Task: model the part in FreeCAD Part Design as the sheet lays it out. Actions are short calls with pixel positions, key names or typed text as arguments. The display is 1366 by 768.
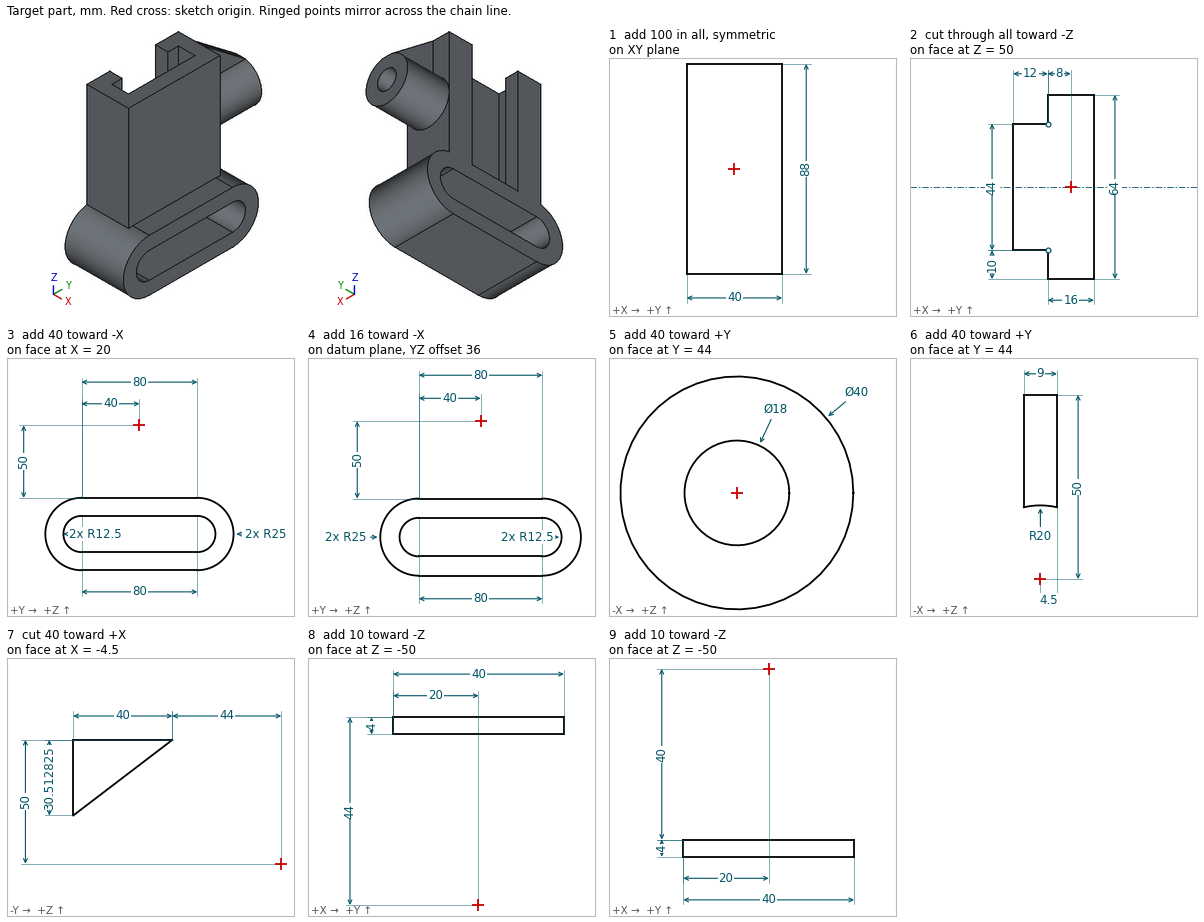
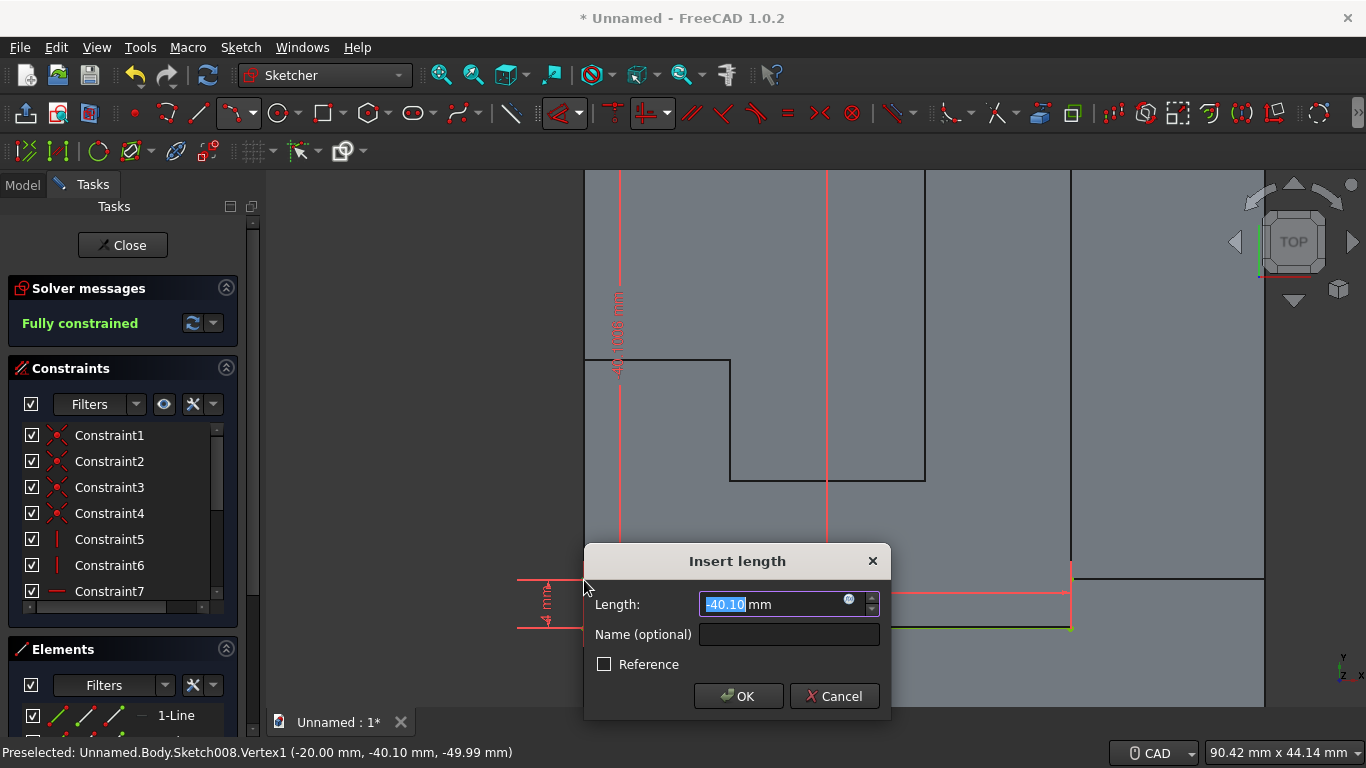
text(-40)
key(Return)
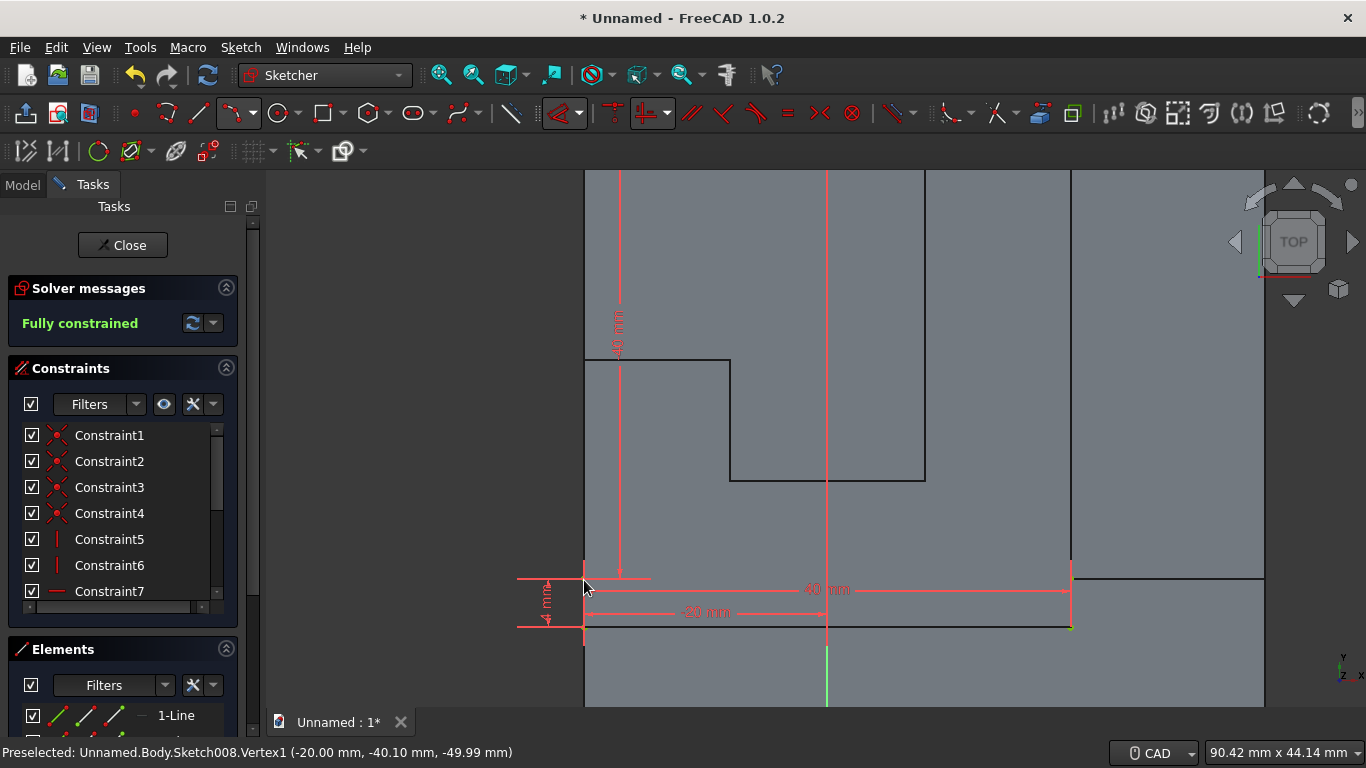
click(123, 245)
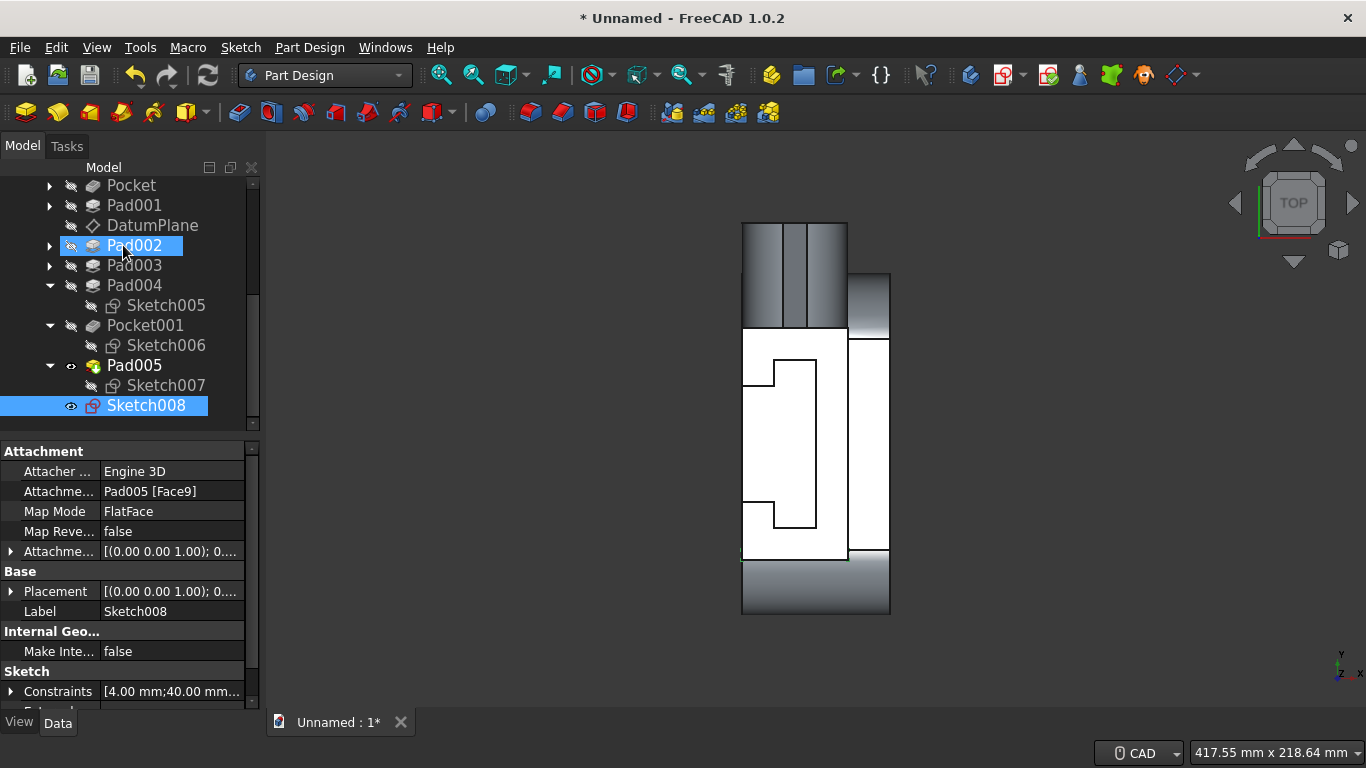
click(26, 112)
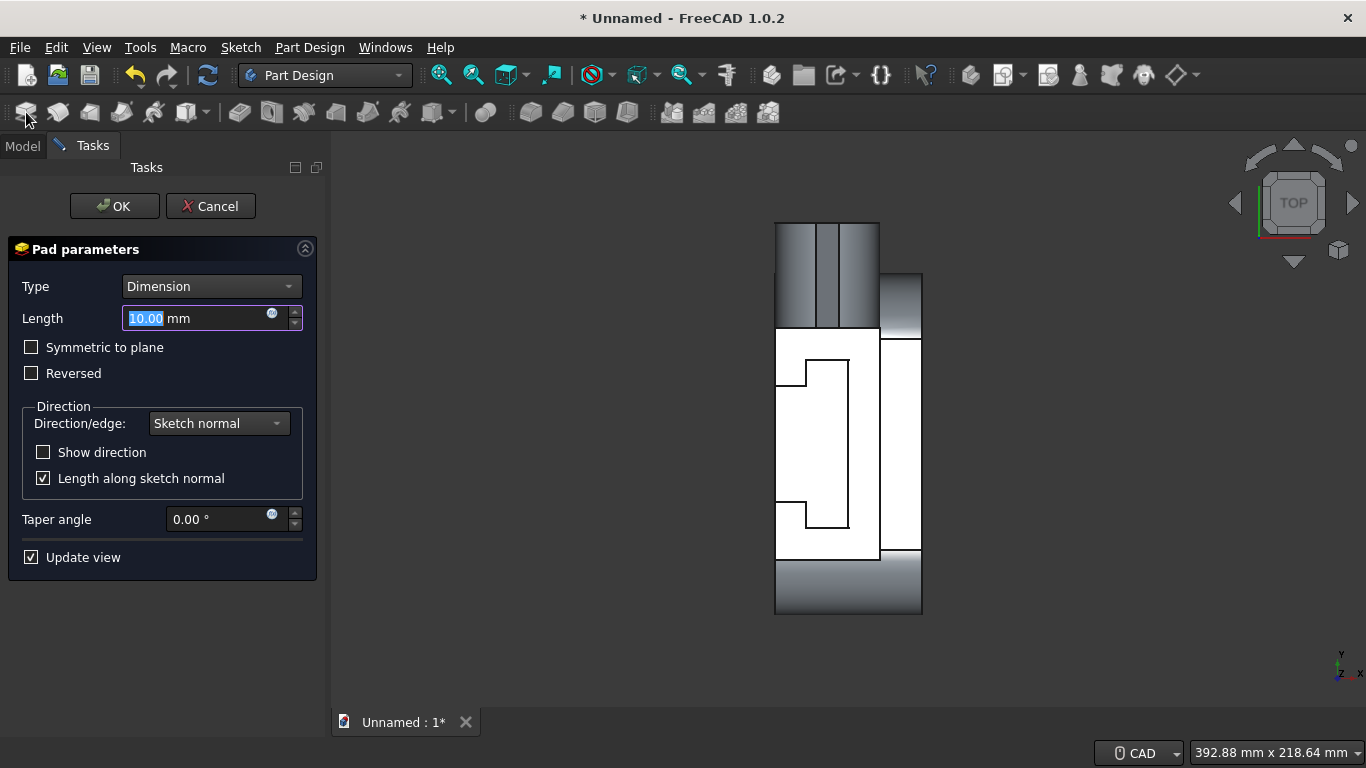
text(10)
key(Tab)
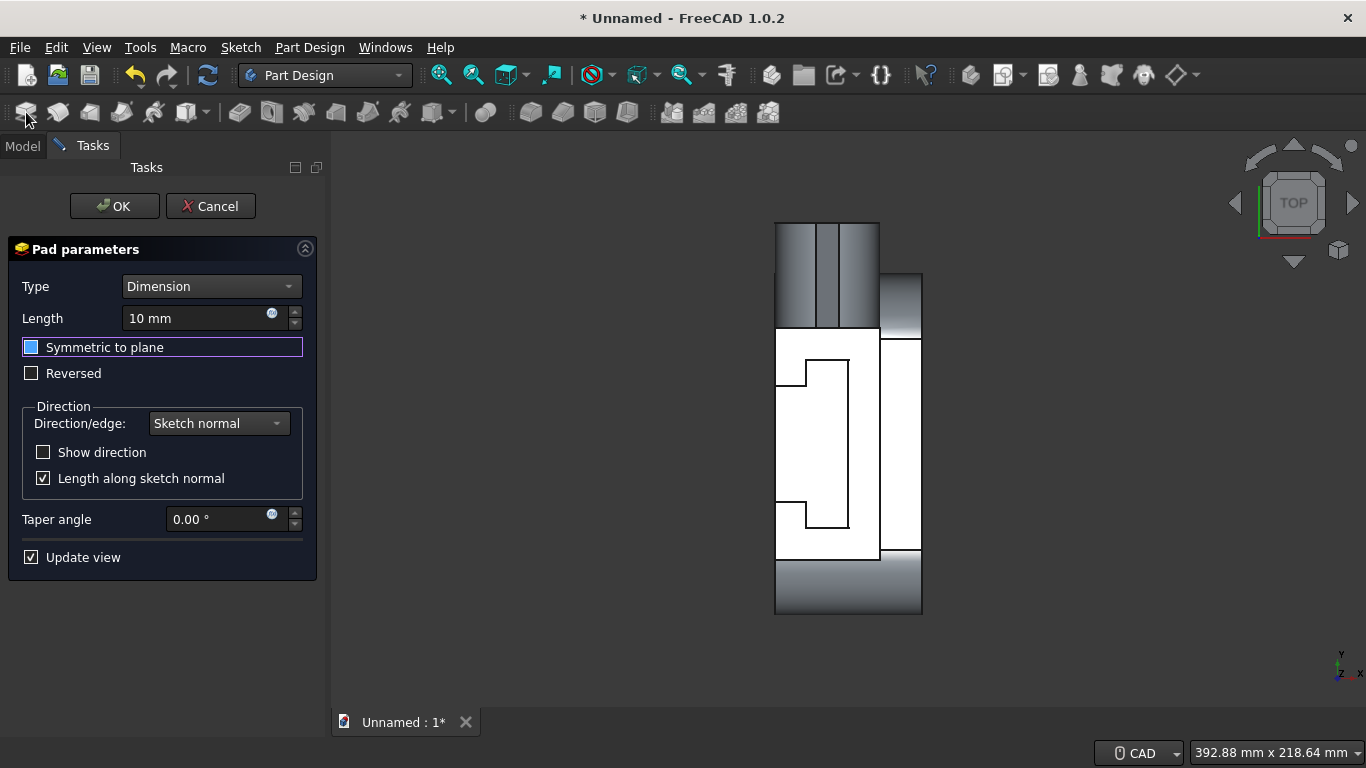
click(30, 373)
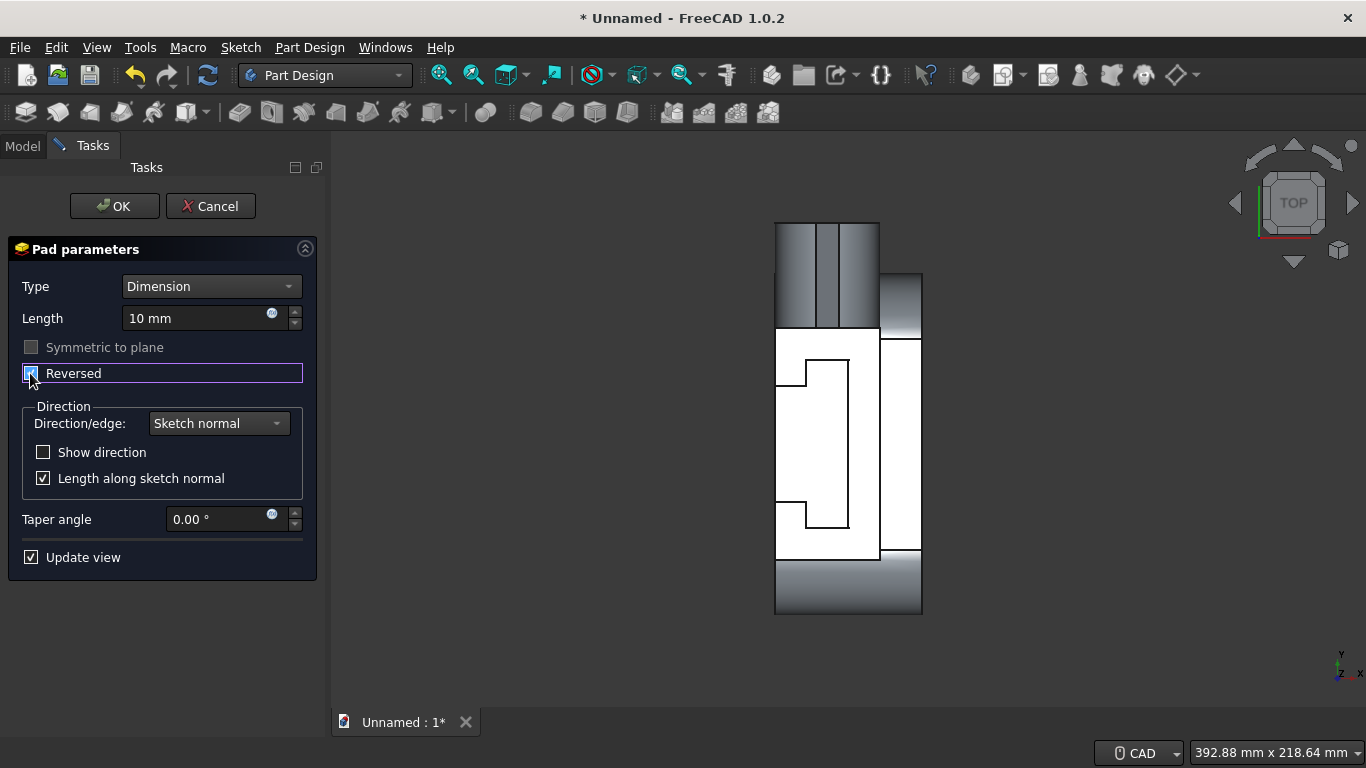
click(115, 206)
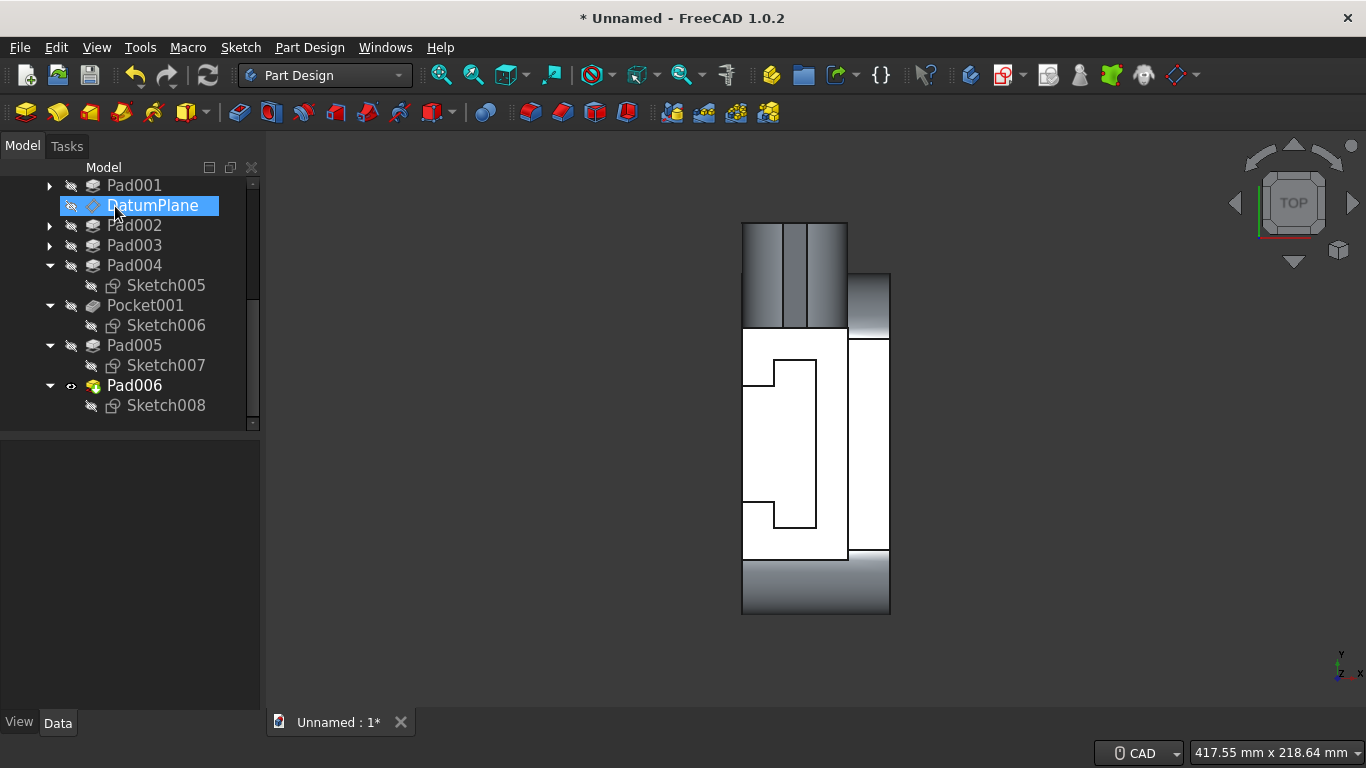
key(0)